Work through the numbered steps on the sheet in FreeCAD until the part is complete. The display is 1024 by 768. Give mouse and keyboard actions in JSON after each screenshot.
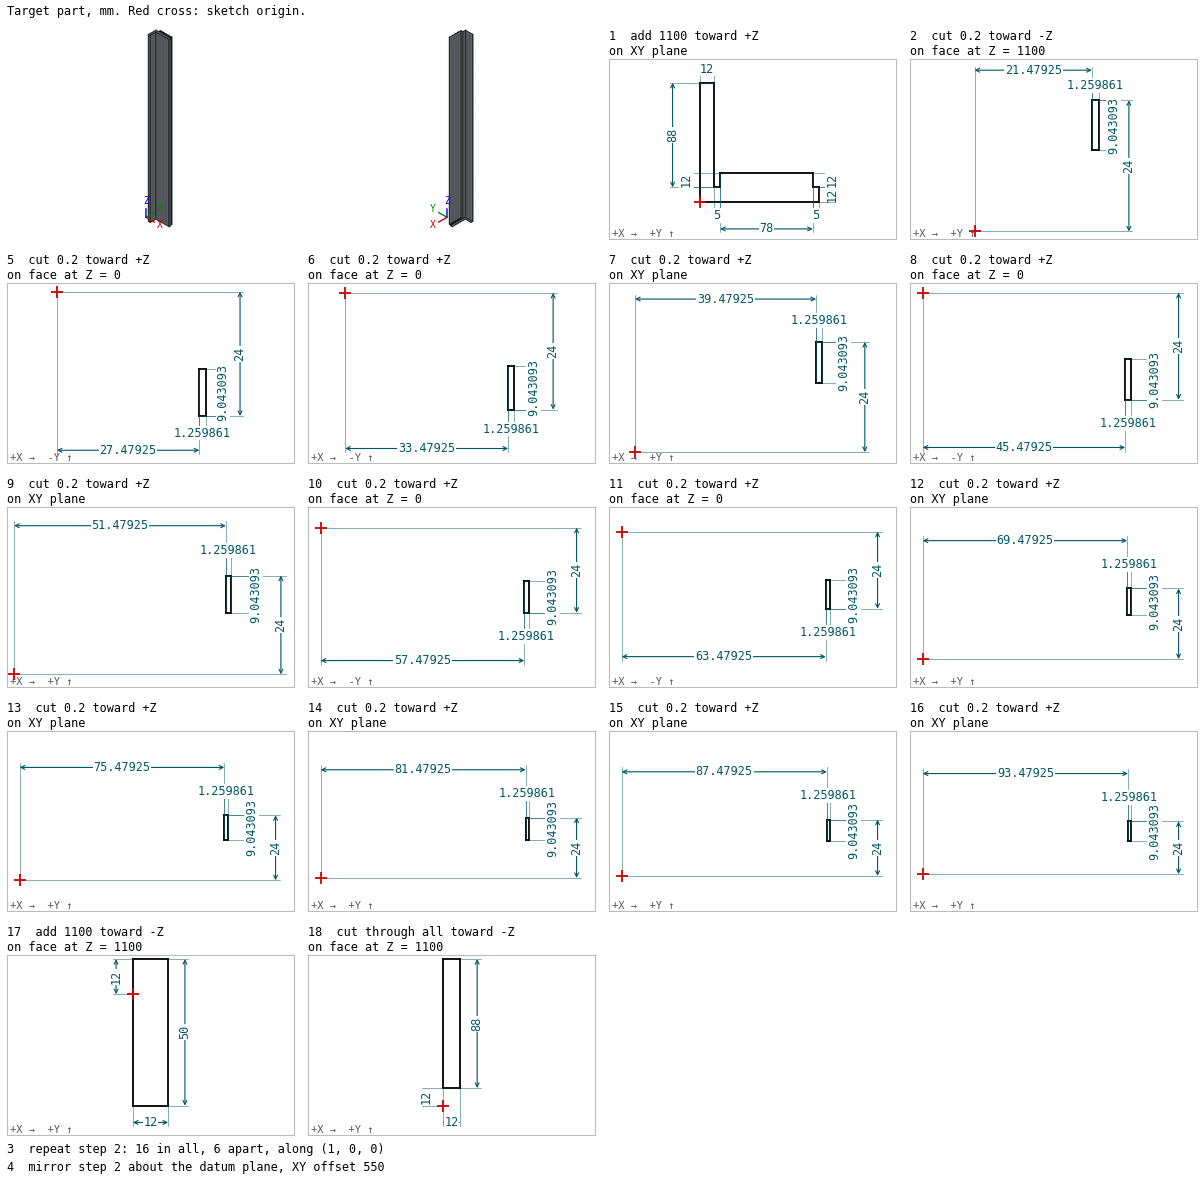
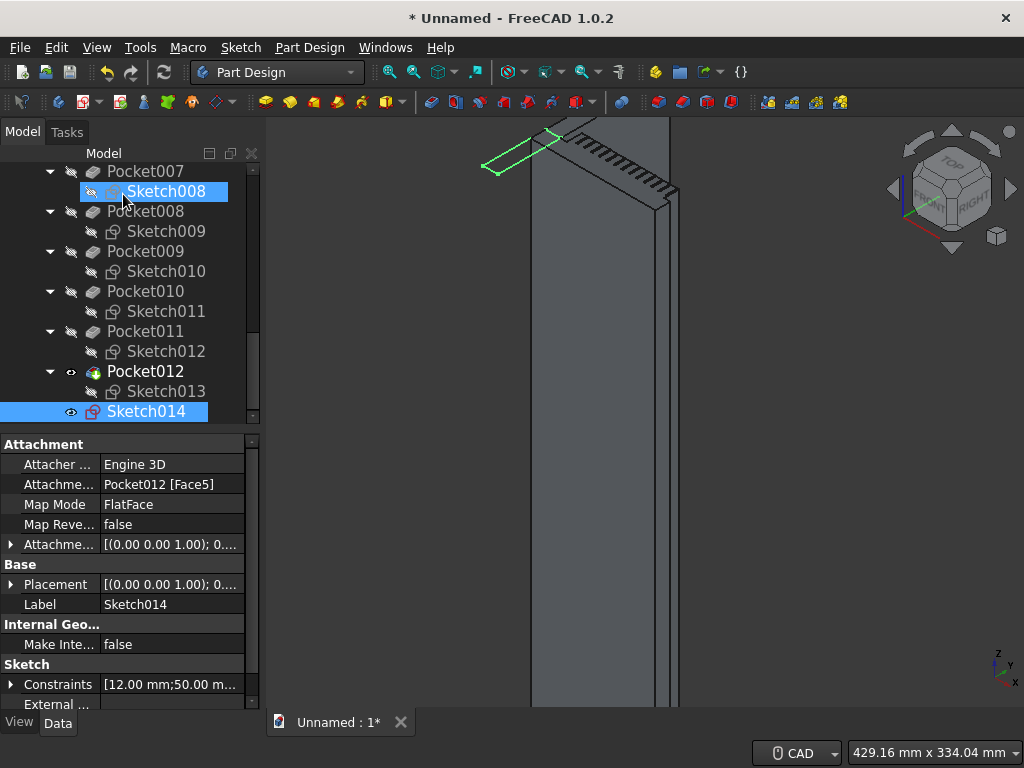
{"action": "left_click", "coordinate": [266, 102]}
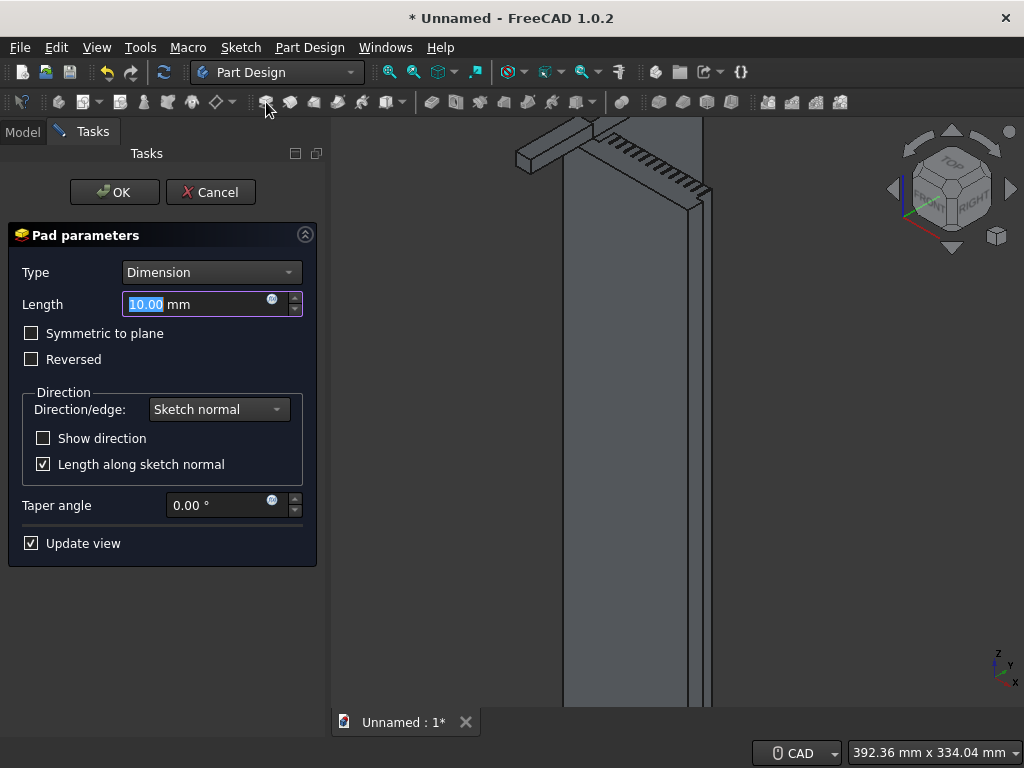
{"action": "type", "text": "1100"}
{"action": "key", "text": "Tab"}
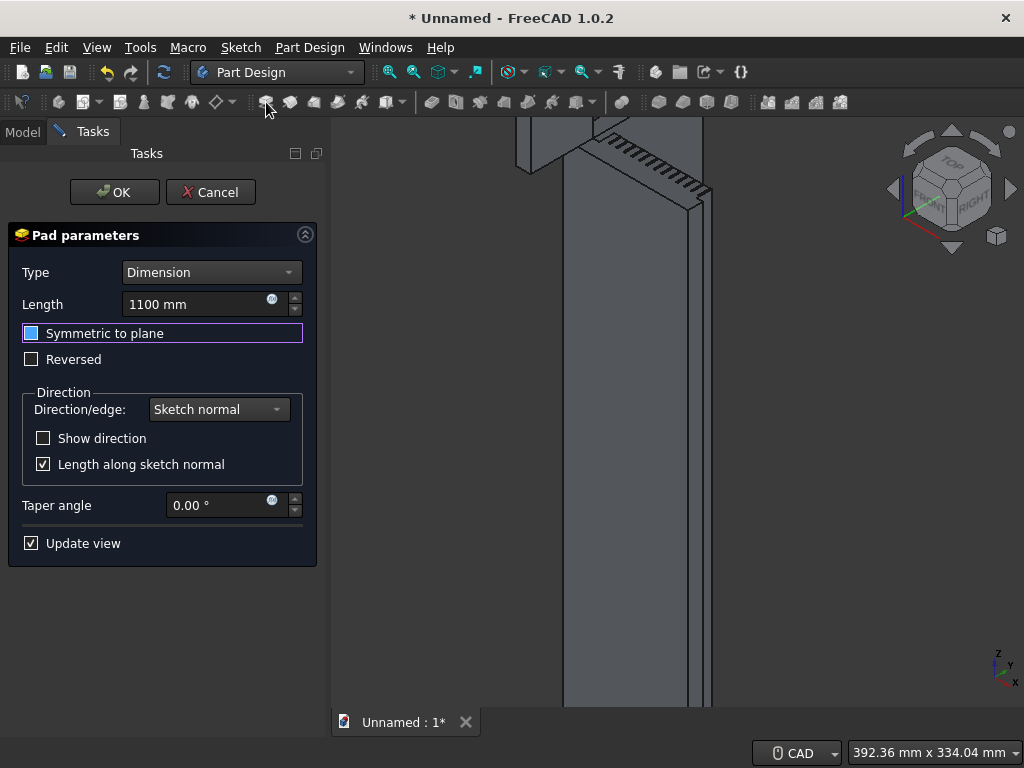
{"action": "left_click", "coordinate": [30, 359]}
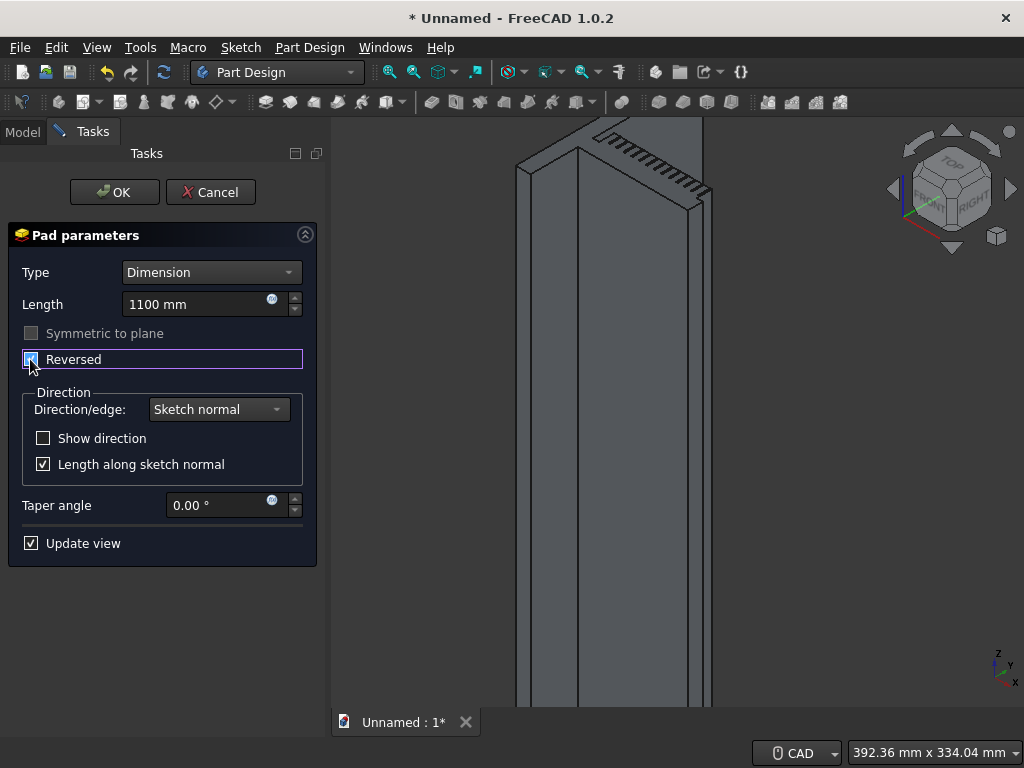
{"action": "left_click", "coordinate": [115, 192]}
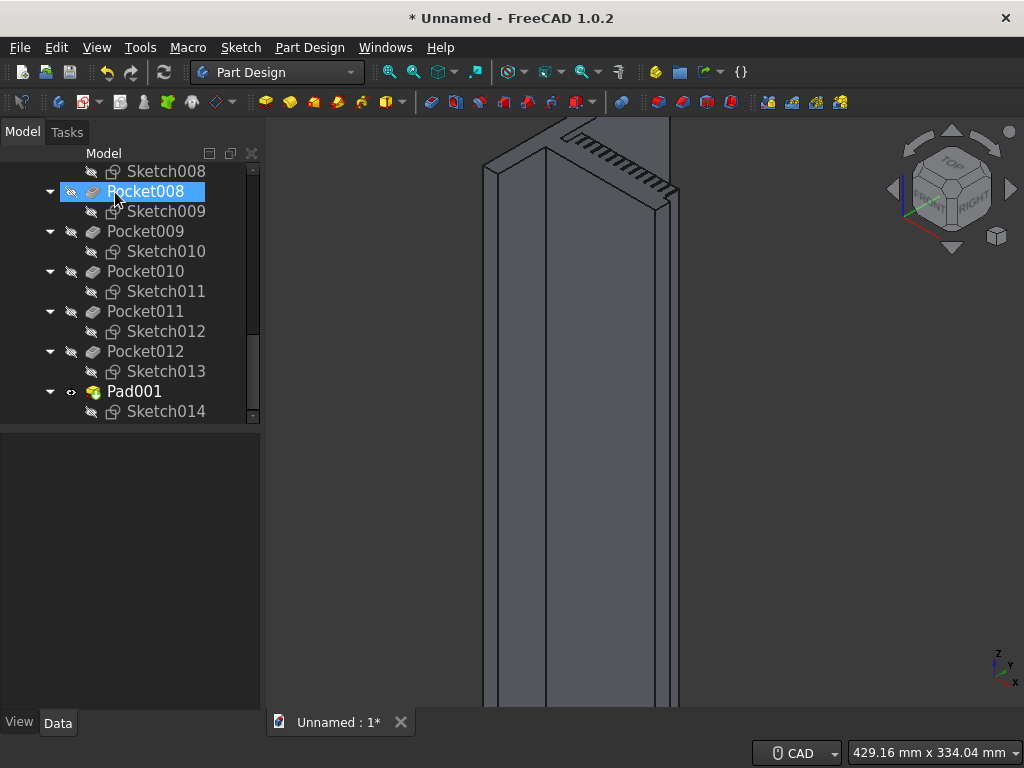
{"action": "left_click", "coordinate": [390, 72]}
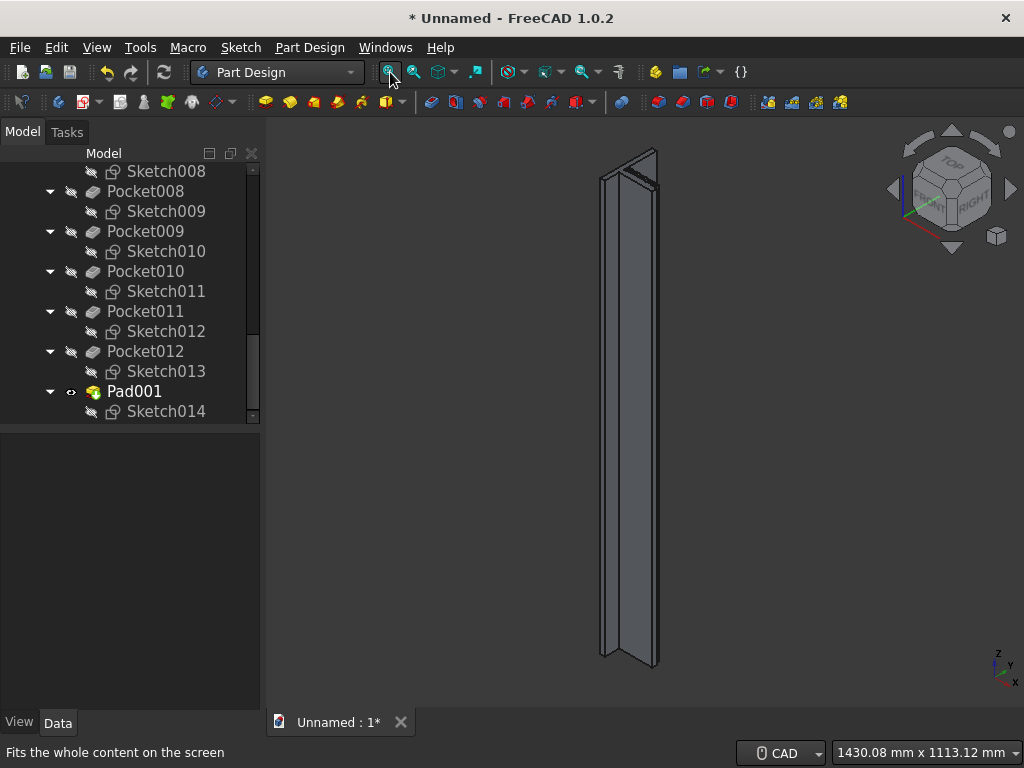
{"action": "scroll", "coordinate": [622, 168], "scroll_direction": "up", "scroll_amount": 8}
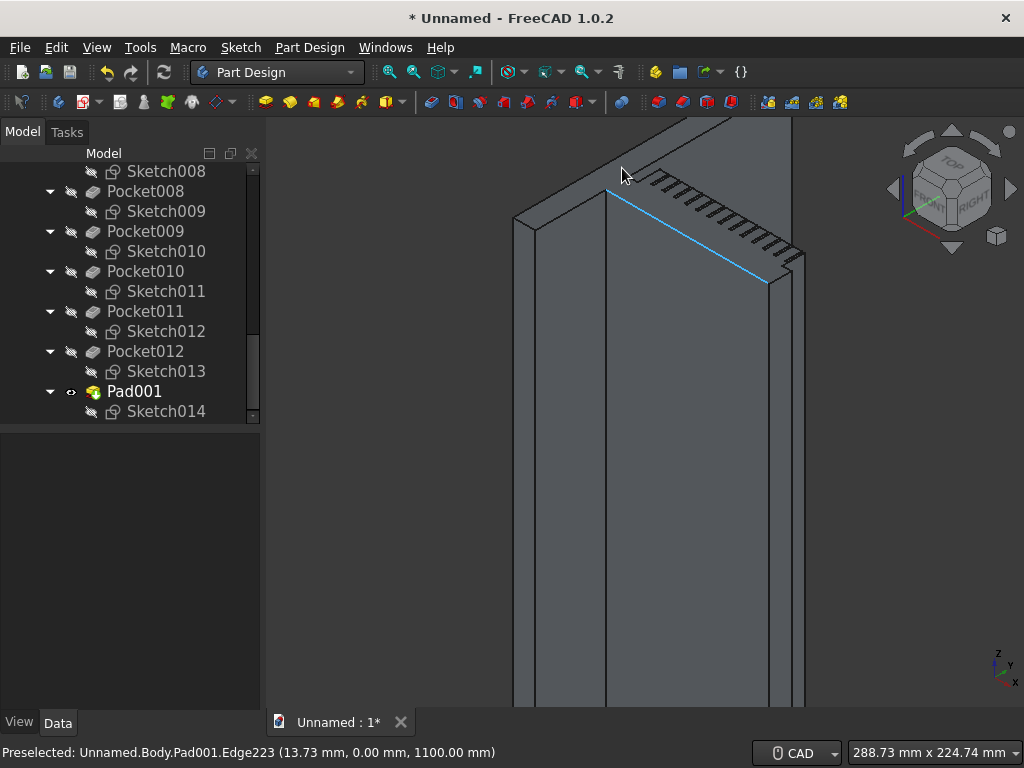
{"action": "left_click", "coordinate": [618, 171]}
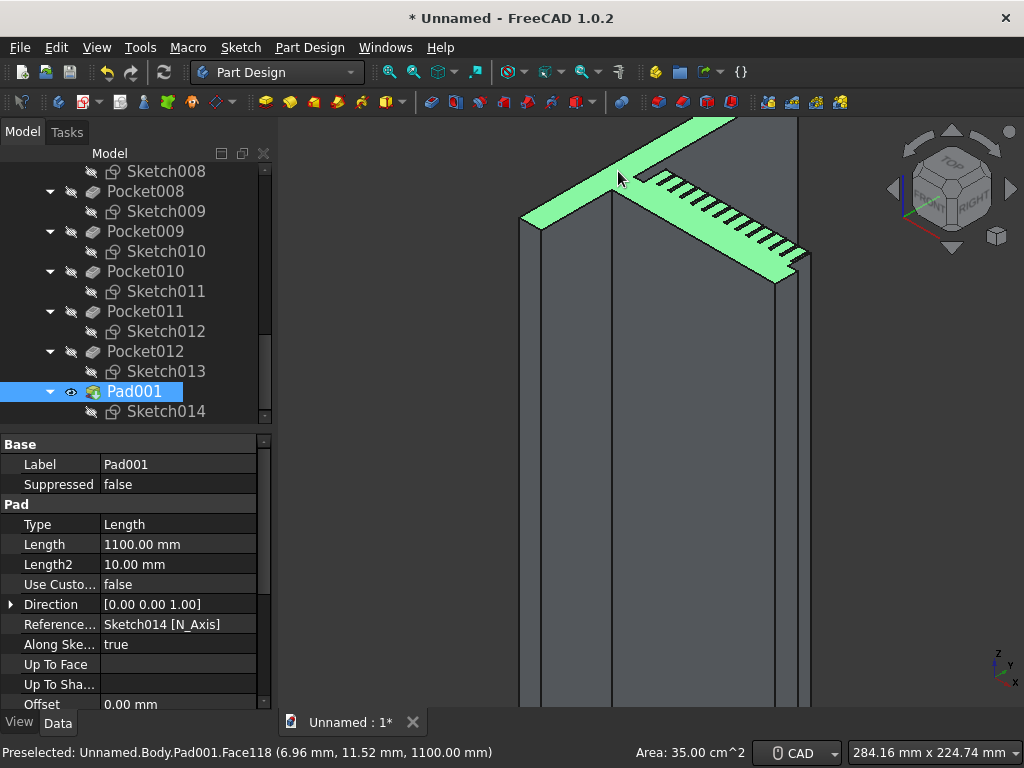
{"action": "left_click", "coordinate": [84, 102]}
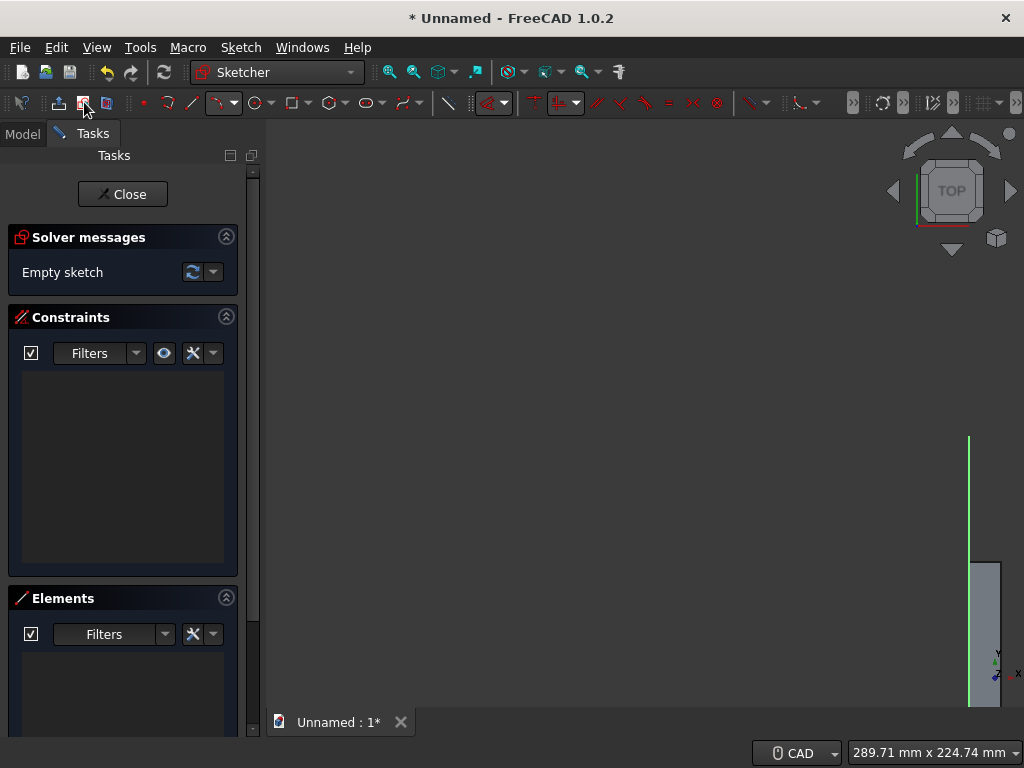
{"action": "scroll", "coordinate": [576, 413], "scroll_direction": "down", "scroll_amount": 5}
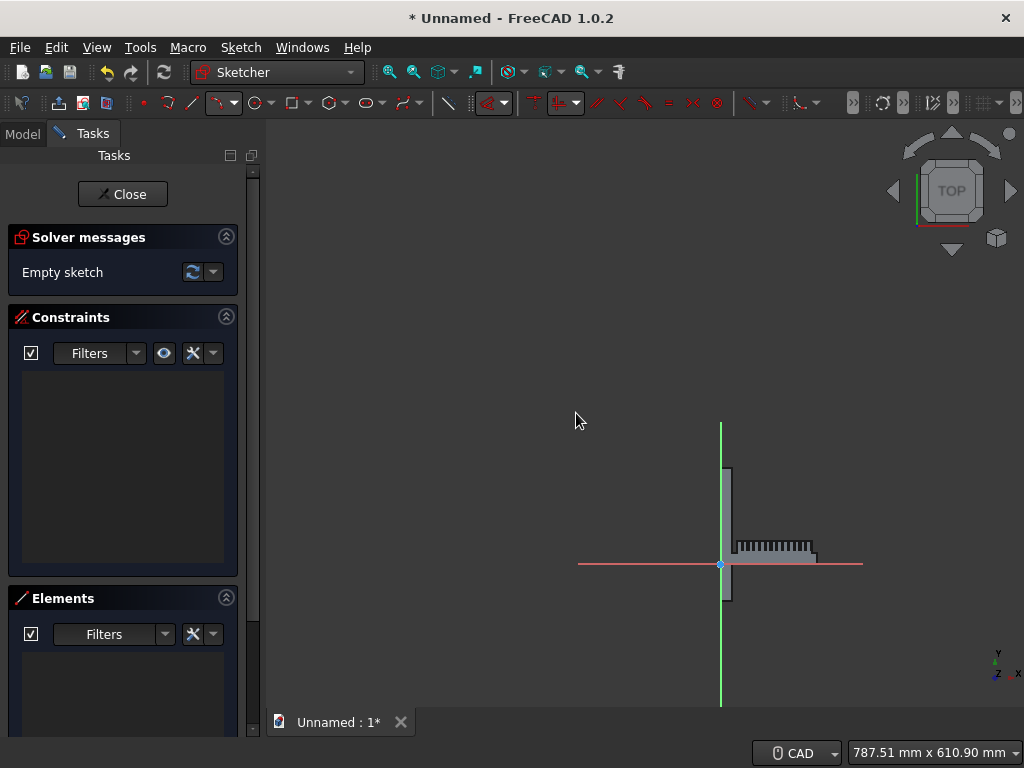
{"action": "scroll", "coordinate": [776, 550], "scroll_direction": "up", "scroll_amount": 7}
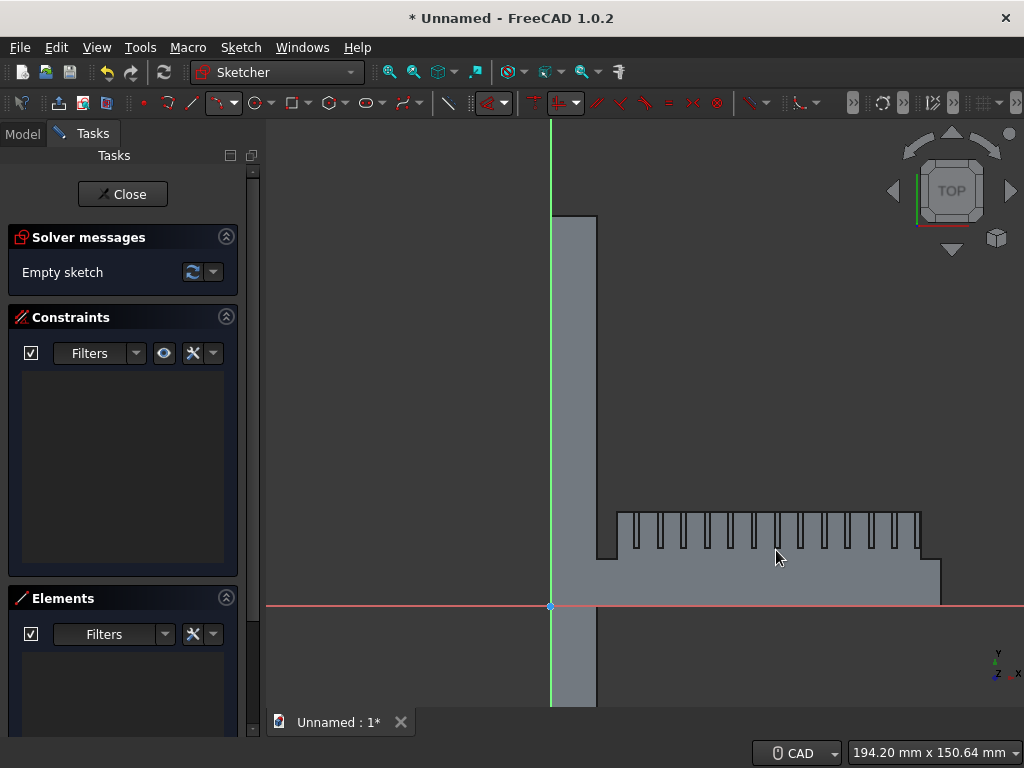
{"action": "left_click", "coordinate": [292, 104]}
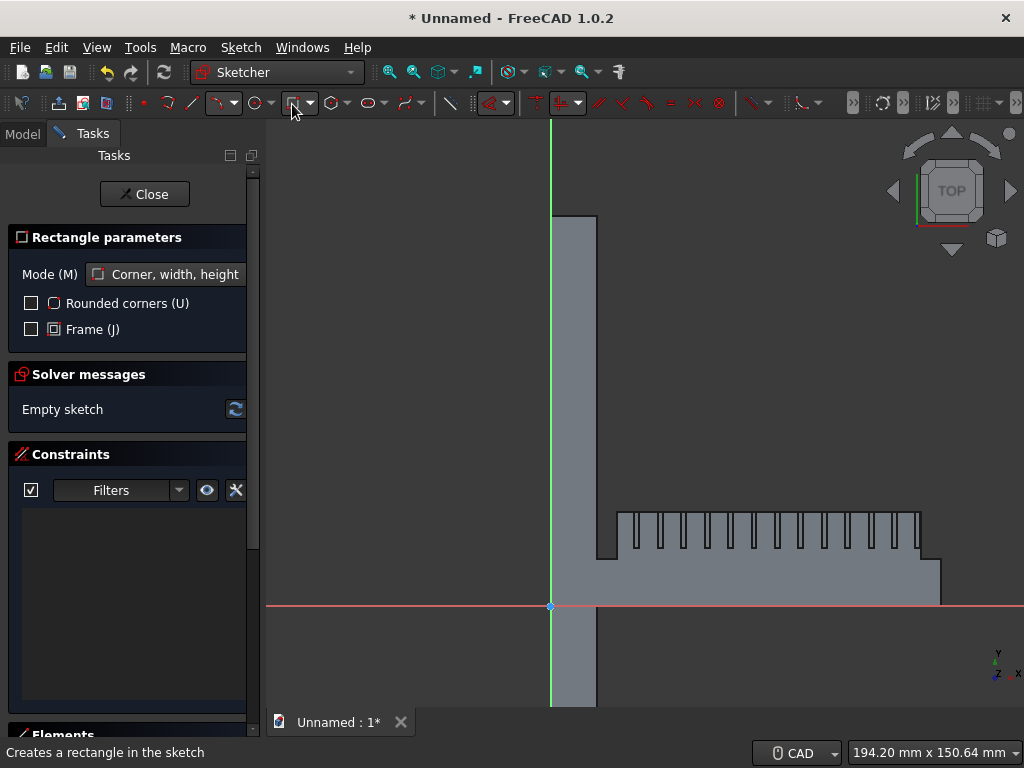
{"action": "left_click", "coordinate": [551, 216]}
{"action": "mouse_move", "coordinate": [597, 559]}